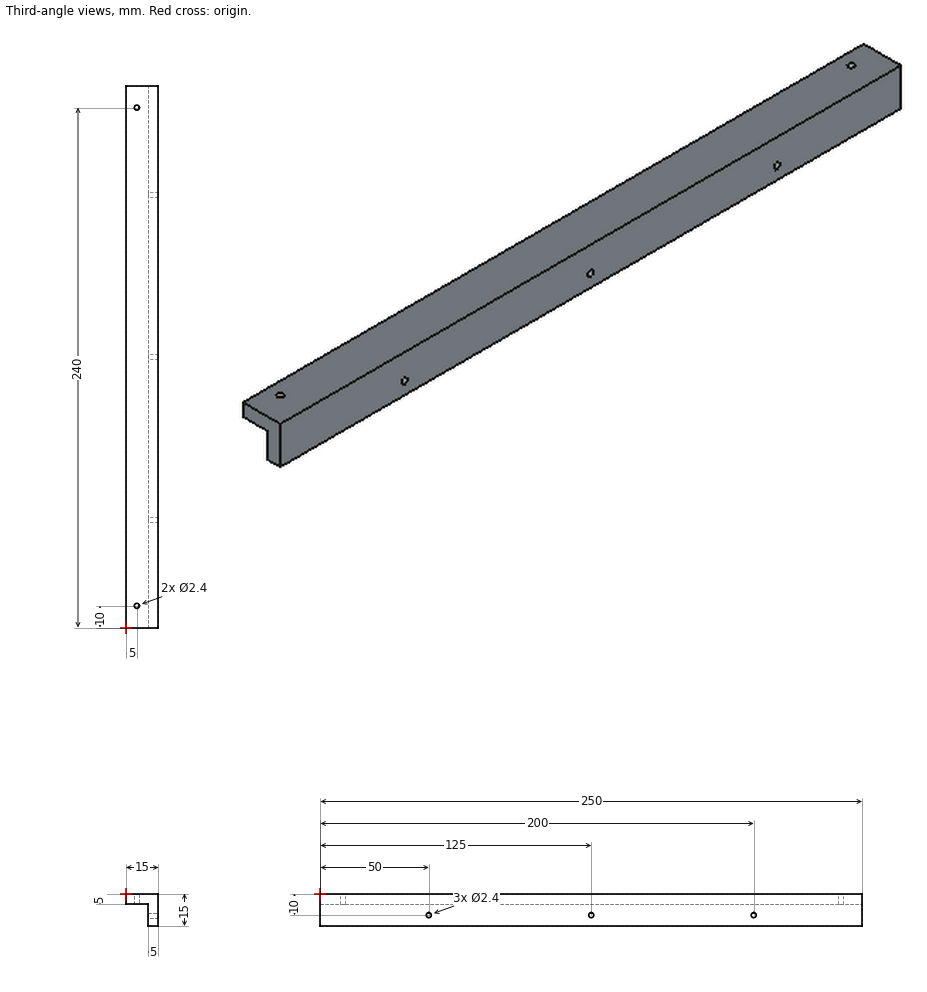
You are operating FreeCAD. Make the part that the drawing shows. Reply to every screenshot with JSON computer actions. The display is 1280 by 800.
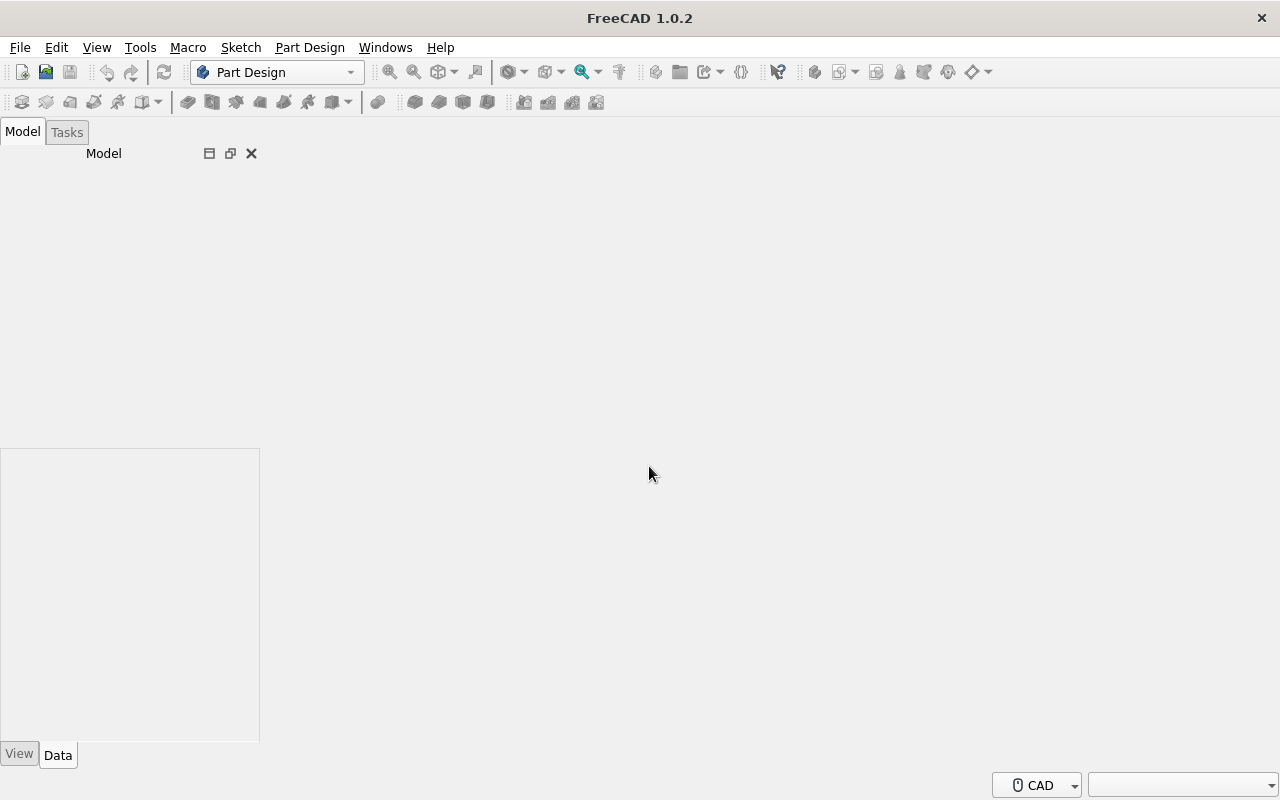
{"action": "left_click", "coordinate": [22, 72]}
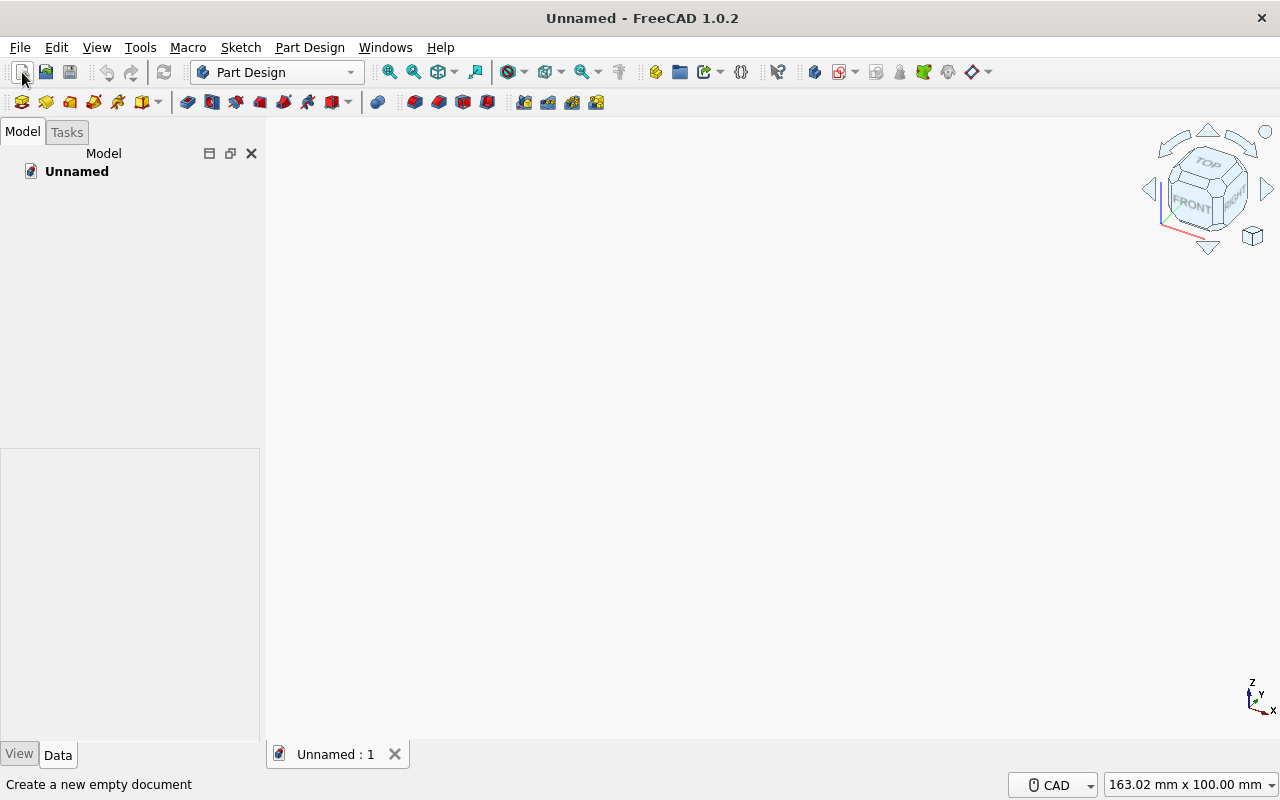
{"action": "left_click", "coordinate": [840, 72]}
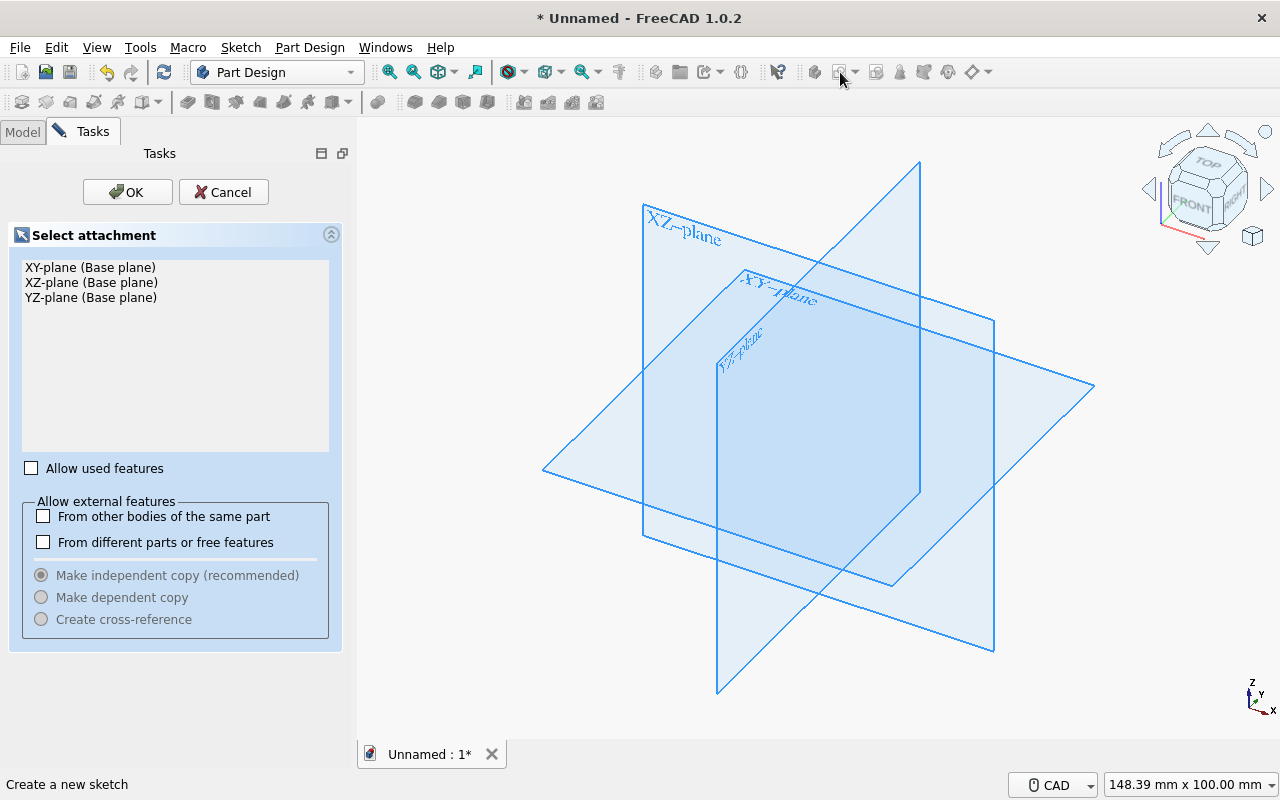
{"action": "left_click", "coordinate": [82, 282]}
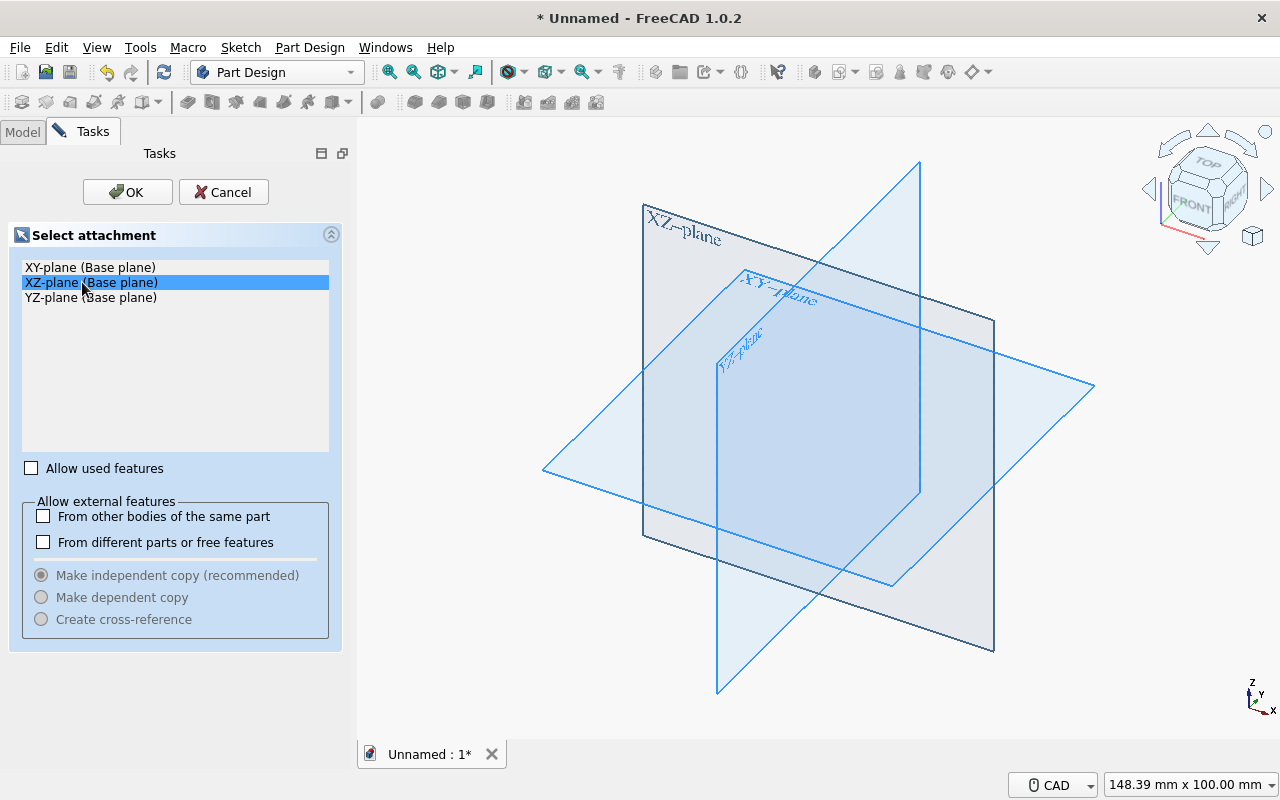
{"action": "left_click", "coordinate": [128, 192]}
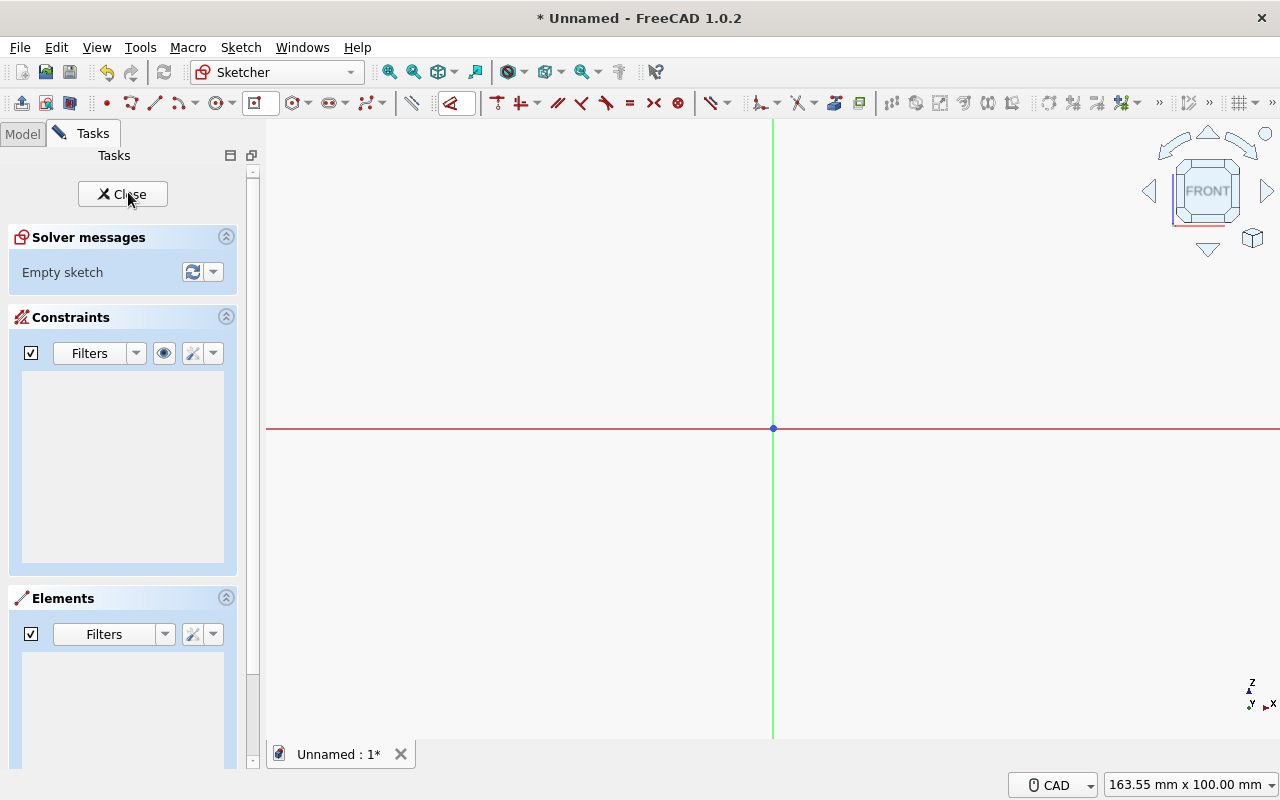
{"action": "scroll", "coordinate": [857, 491], "scroll_direction": "up", "scroll_amount": 7}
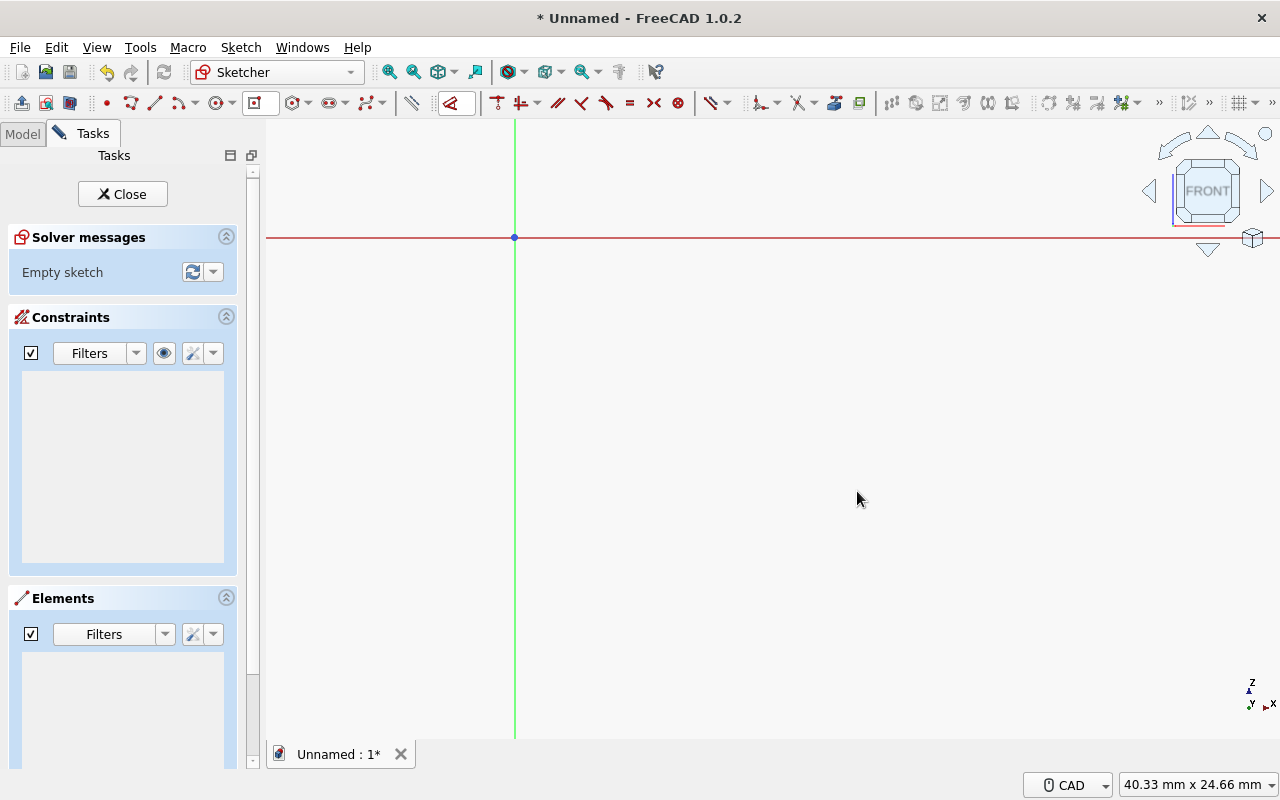
{"action": "left_click", "coordinate": [132, 104]}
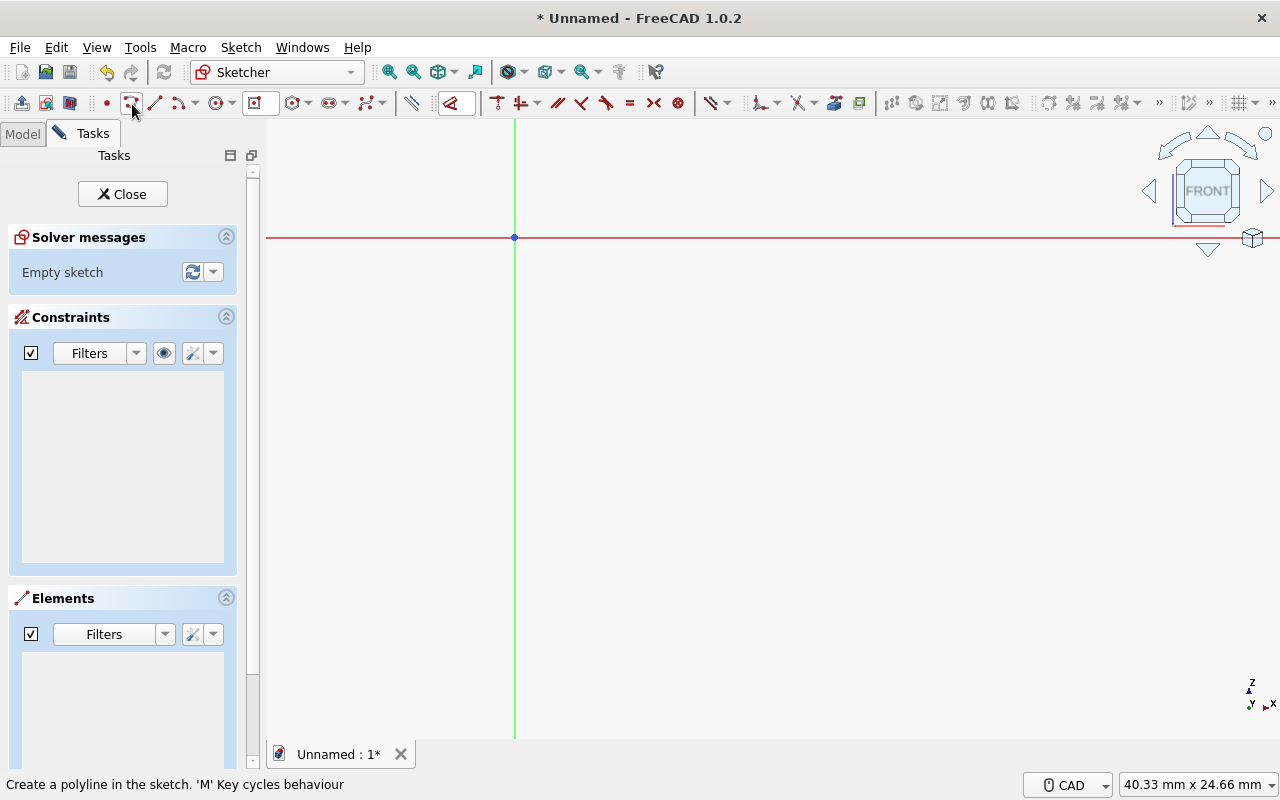
{"action": "left_click", "coordinate": [515, 238]}
{"action": "left_click", "coordinate": [892, 247]}
{"action": "left_click", "coordinate": [892, 615]}
{"action": "left_click", "coordinate": [766, 615]}
{"action": "left_click", "coordinate": [766, 363]}
{"action": "left_click", "coordinate": [524, 363]}
{"action": "left_click", "coordinate": [515, 238]}
{"action": "key", "text": "Escape"}
{"action": "key", "text": "Escape"}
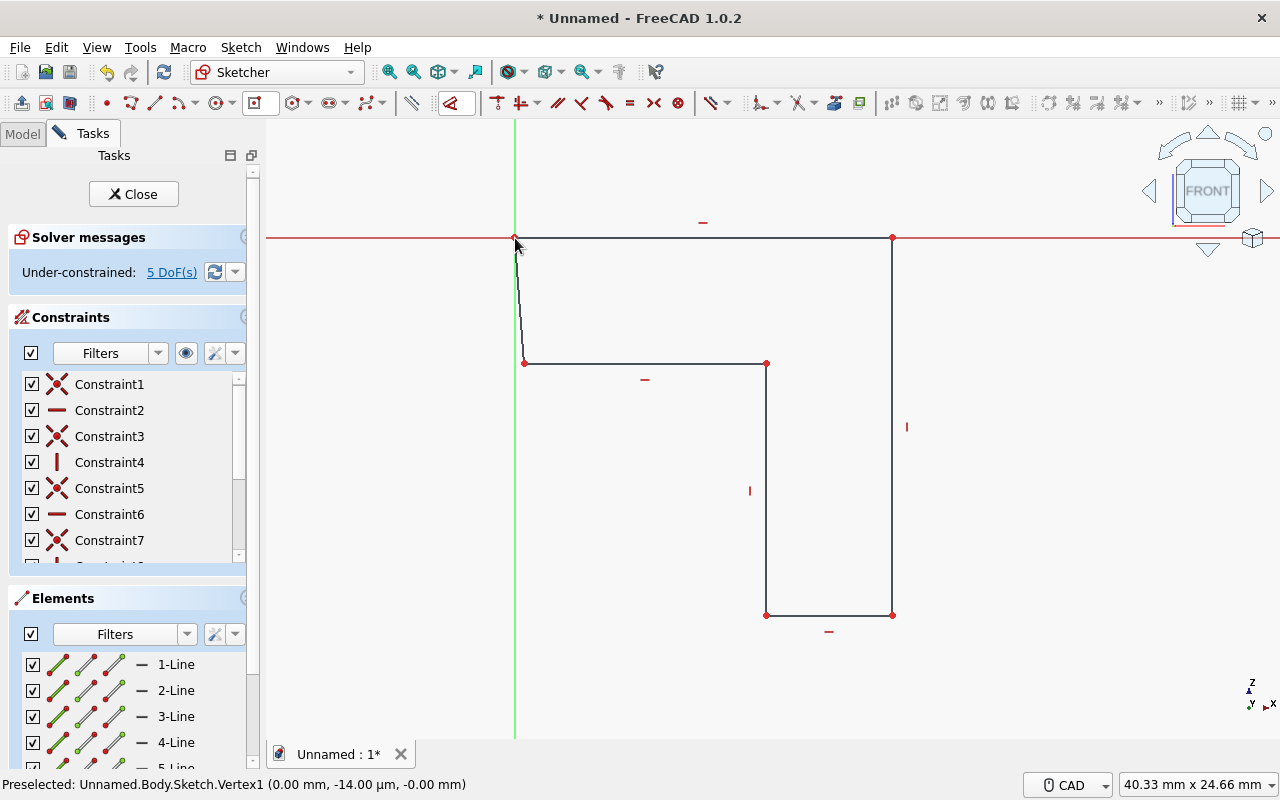
{"action": "left_click", "coordinate": [517, 276]}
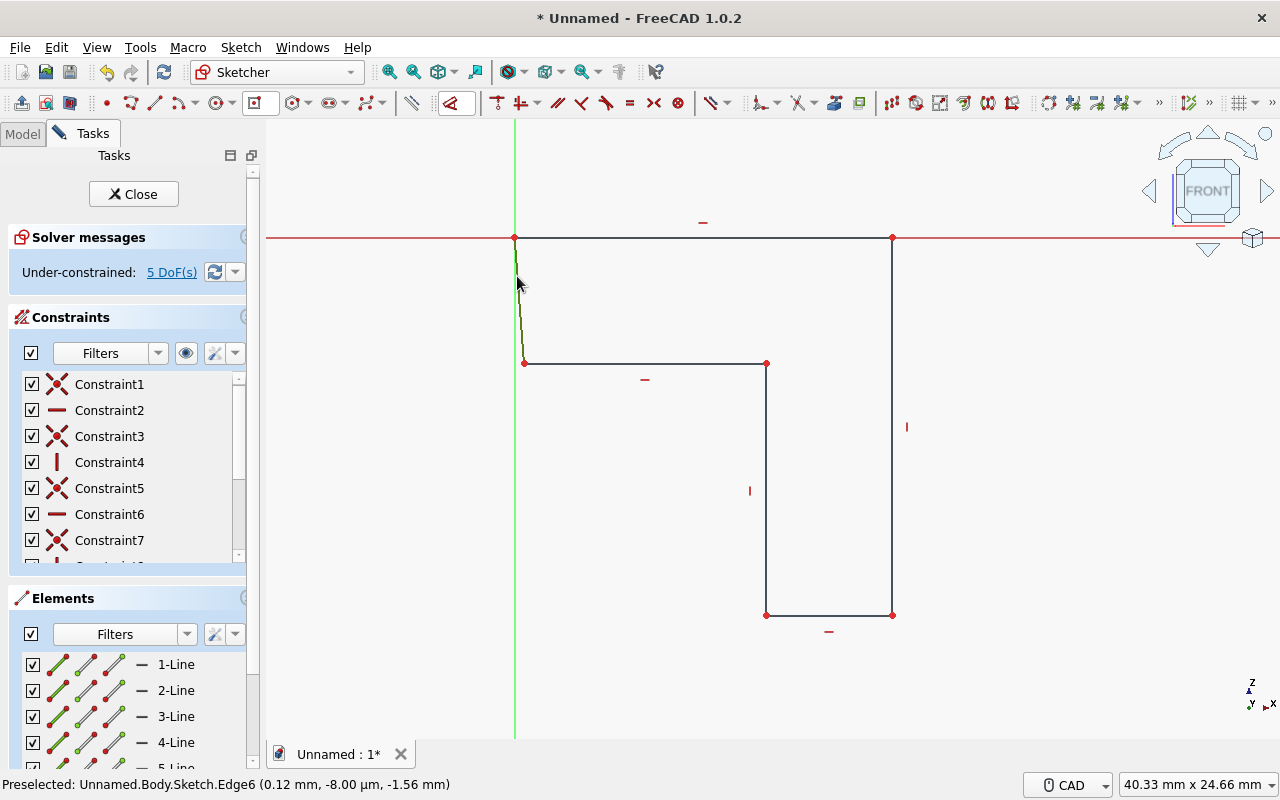
{"action": "key", "text": "v"}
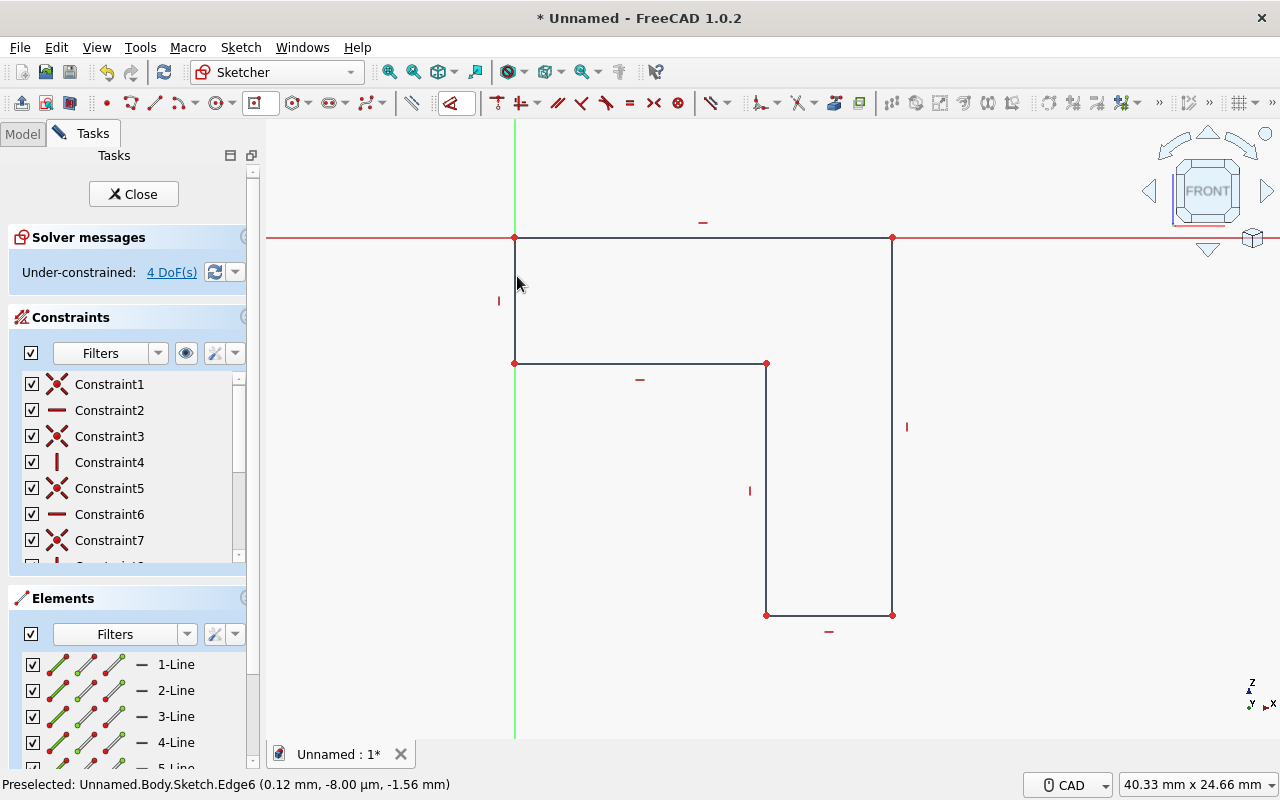
{"action": "key", "text": "d"}